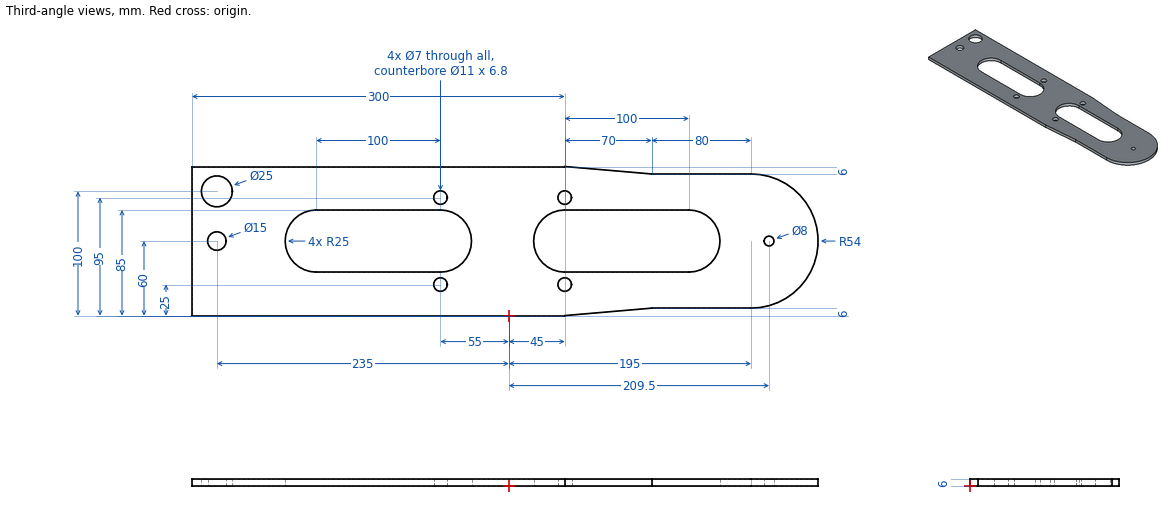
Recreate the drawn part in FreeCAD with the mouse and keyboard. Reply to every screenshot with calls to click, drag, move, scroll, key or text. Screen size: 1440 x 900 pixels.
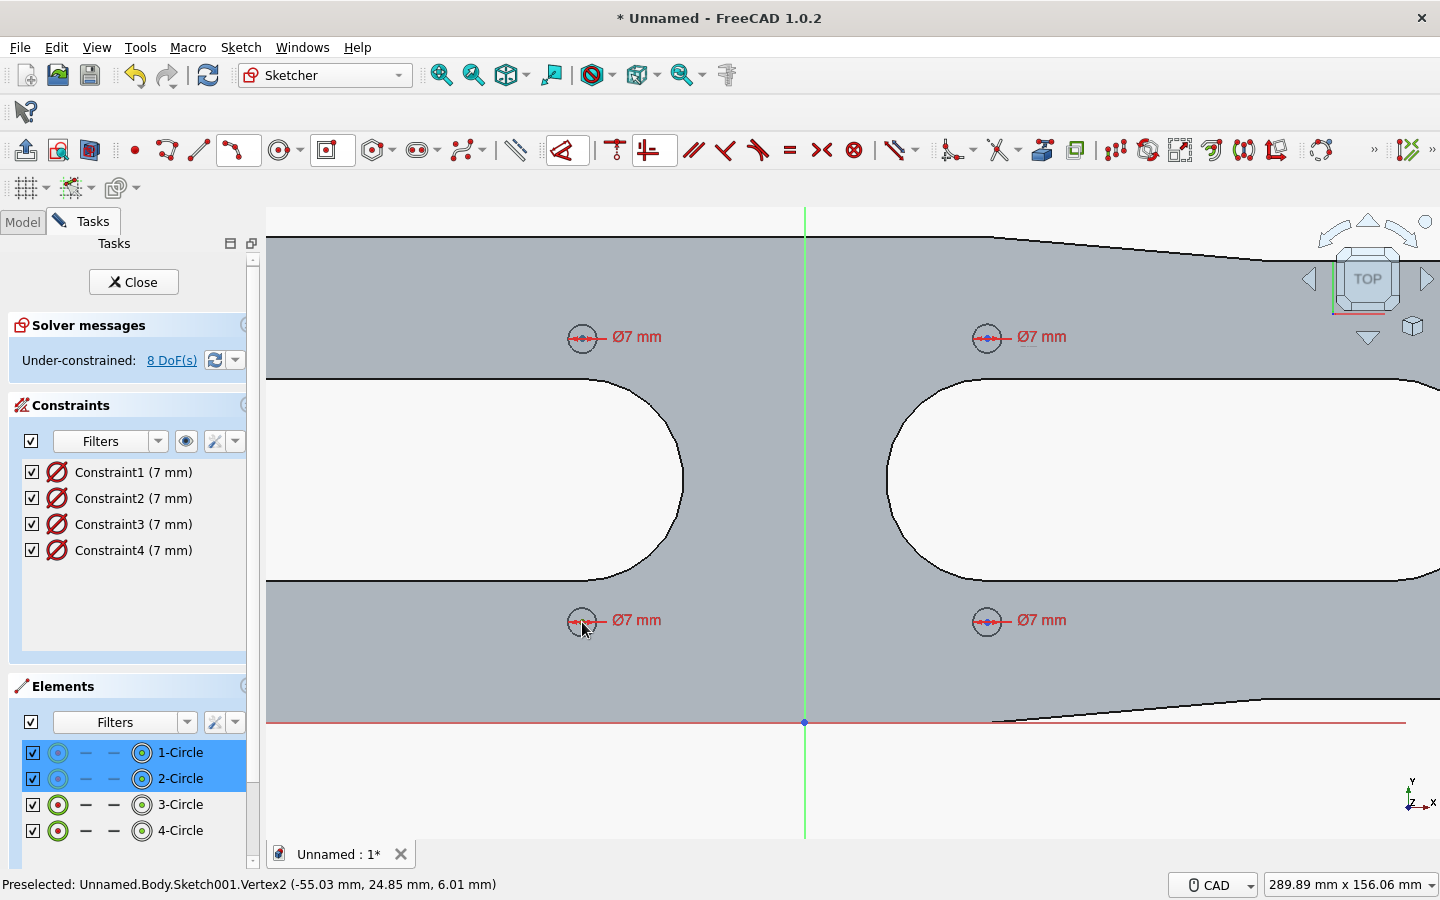
click(672, 150)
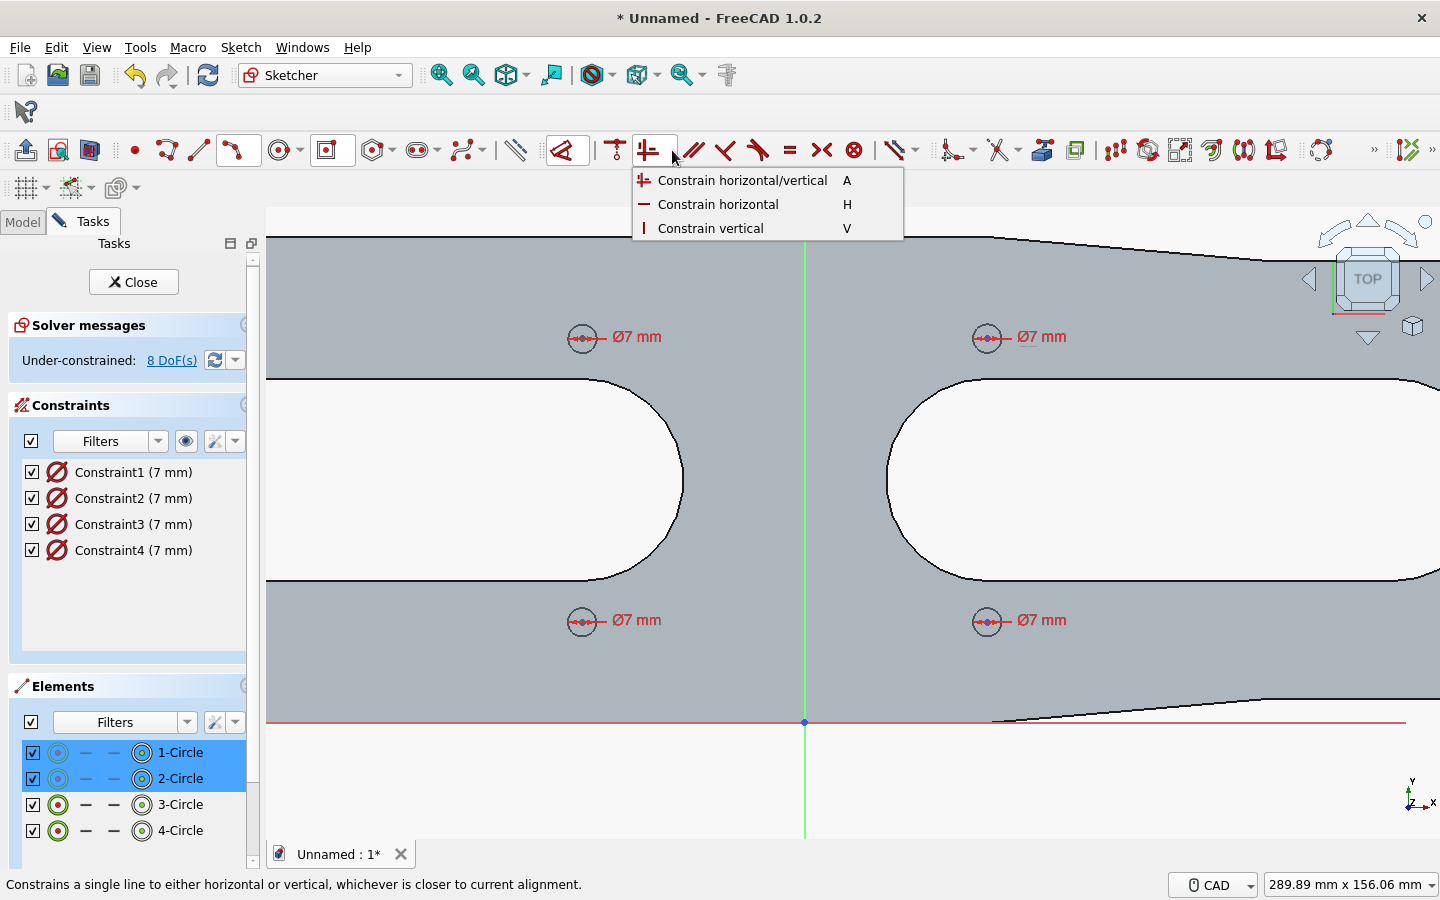
click(768, 228)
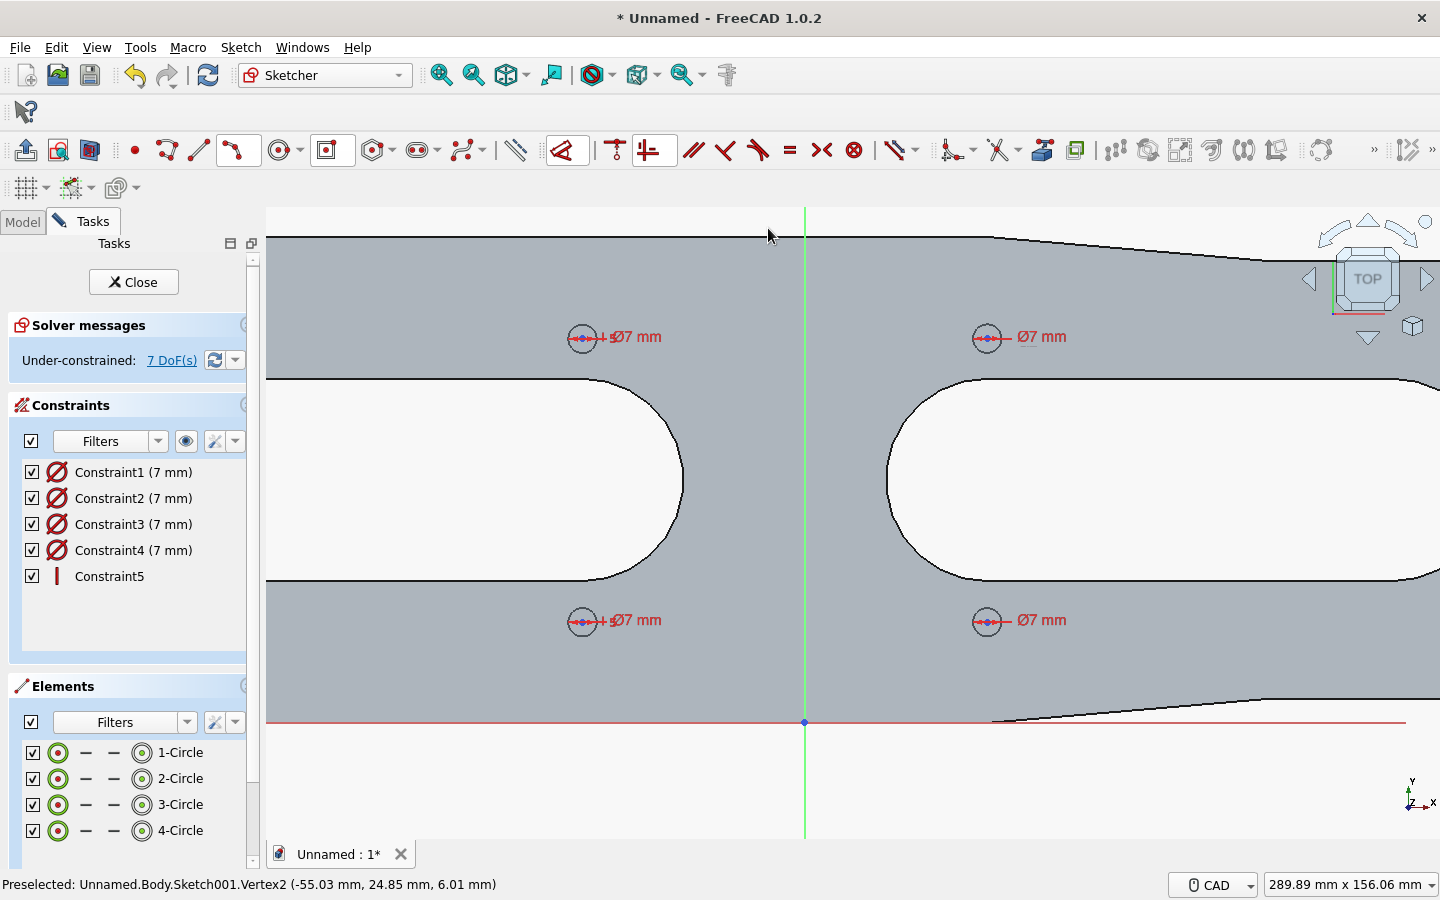
click(582, 339)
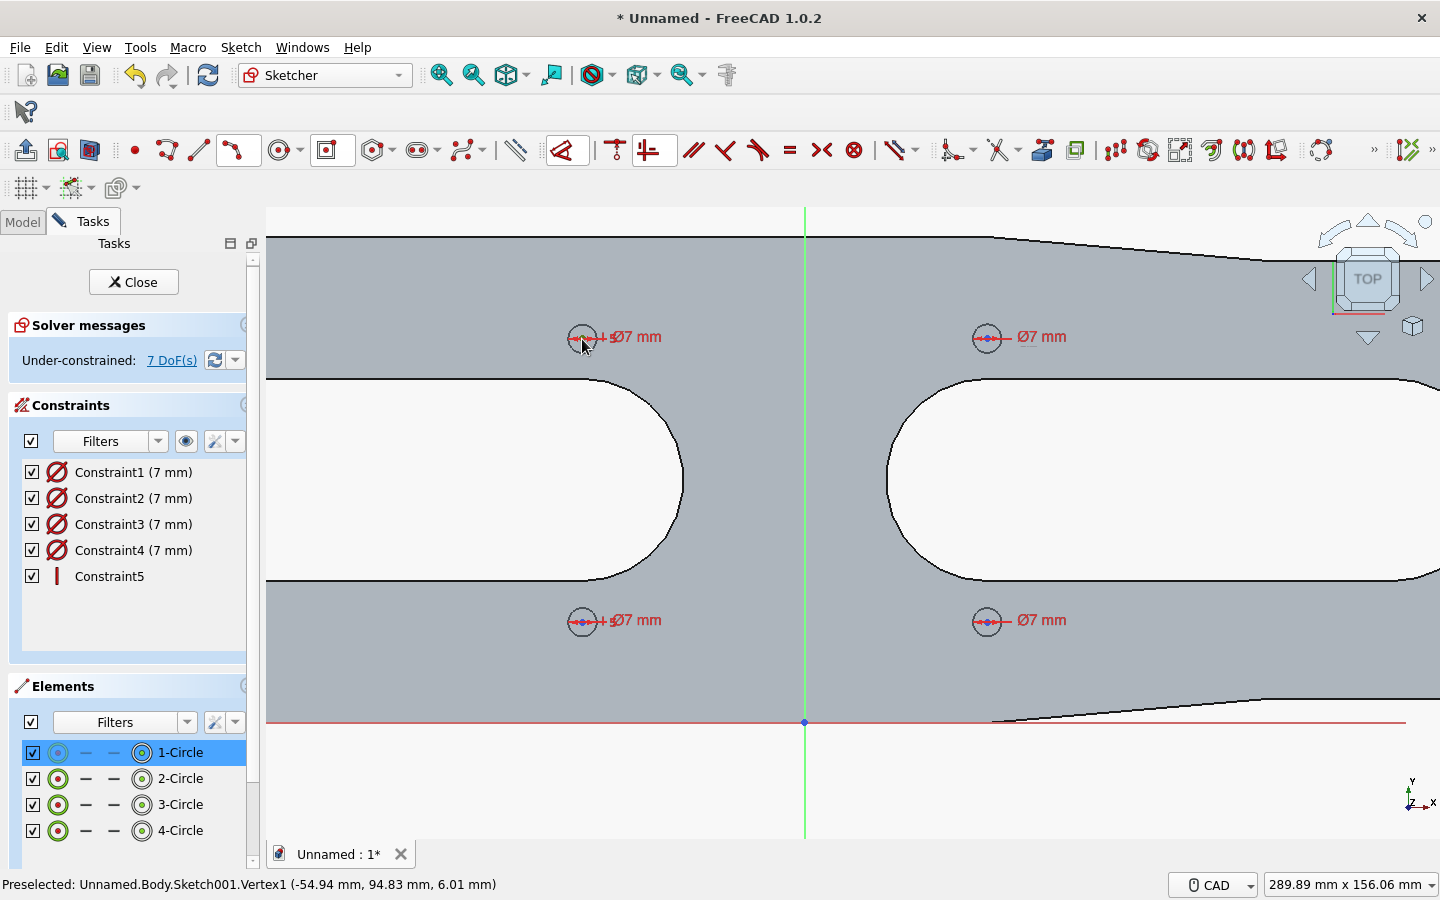
click(987, 339)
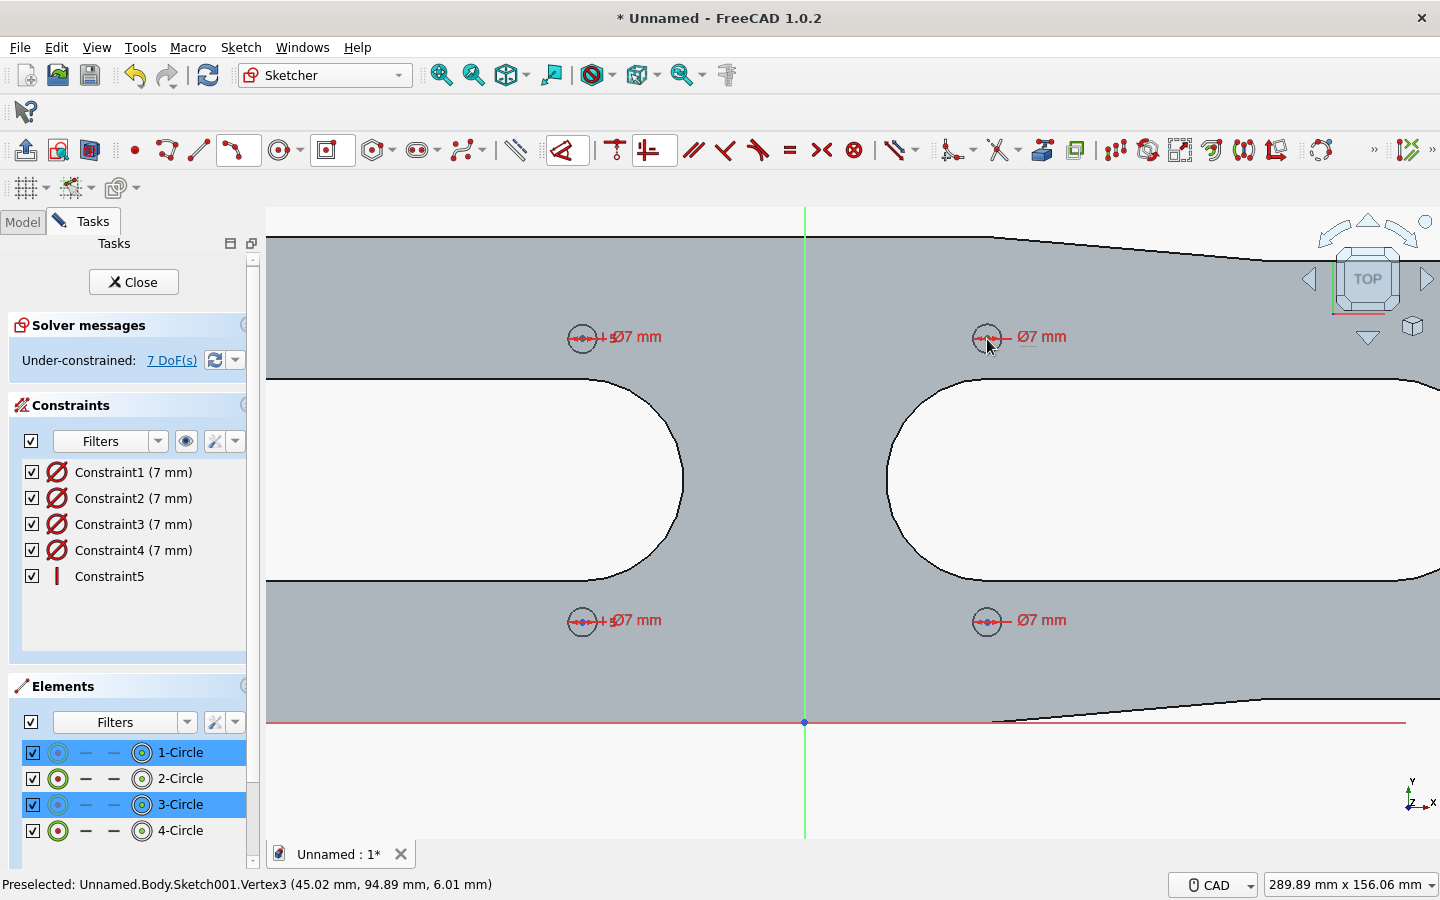
key(h)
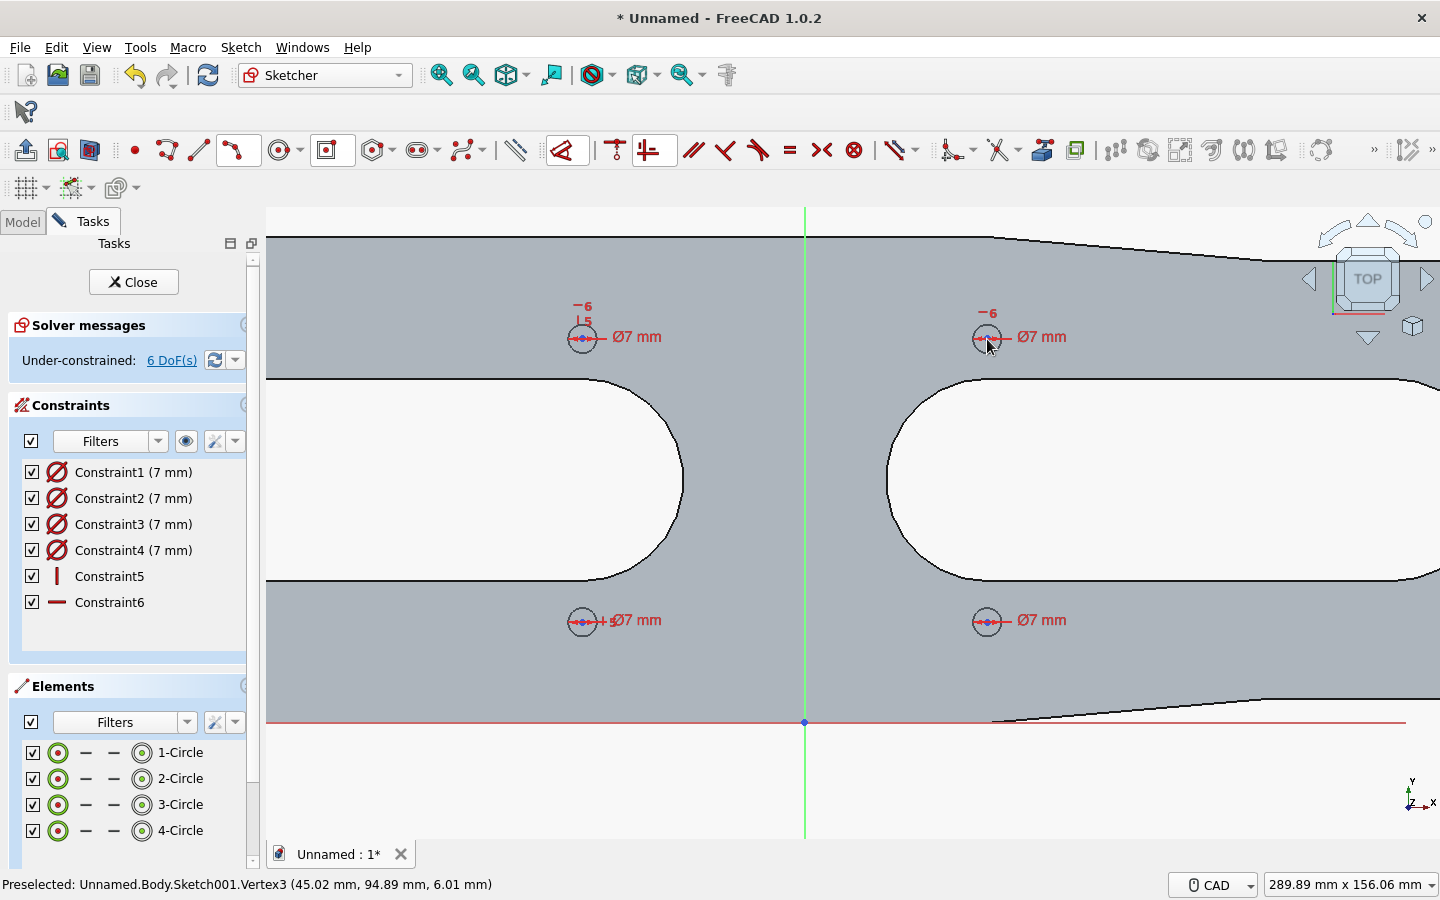
click(987, 339)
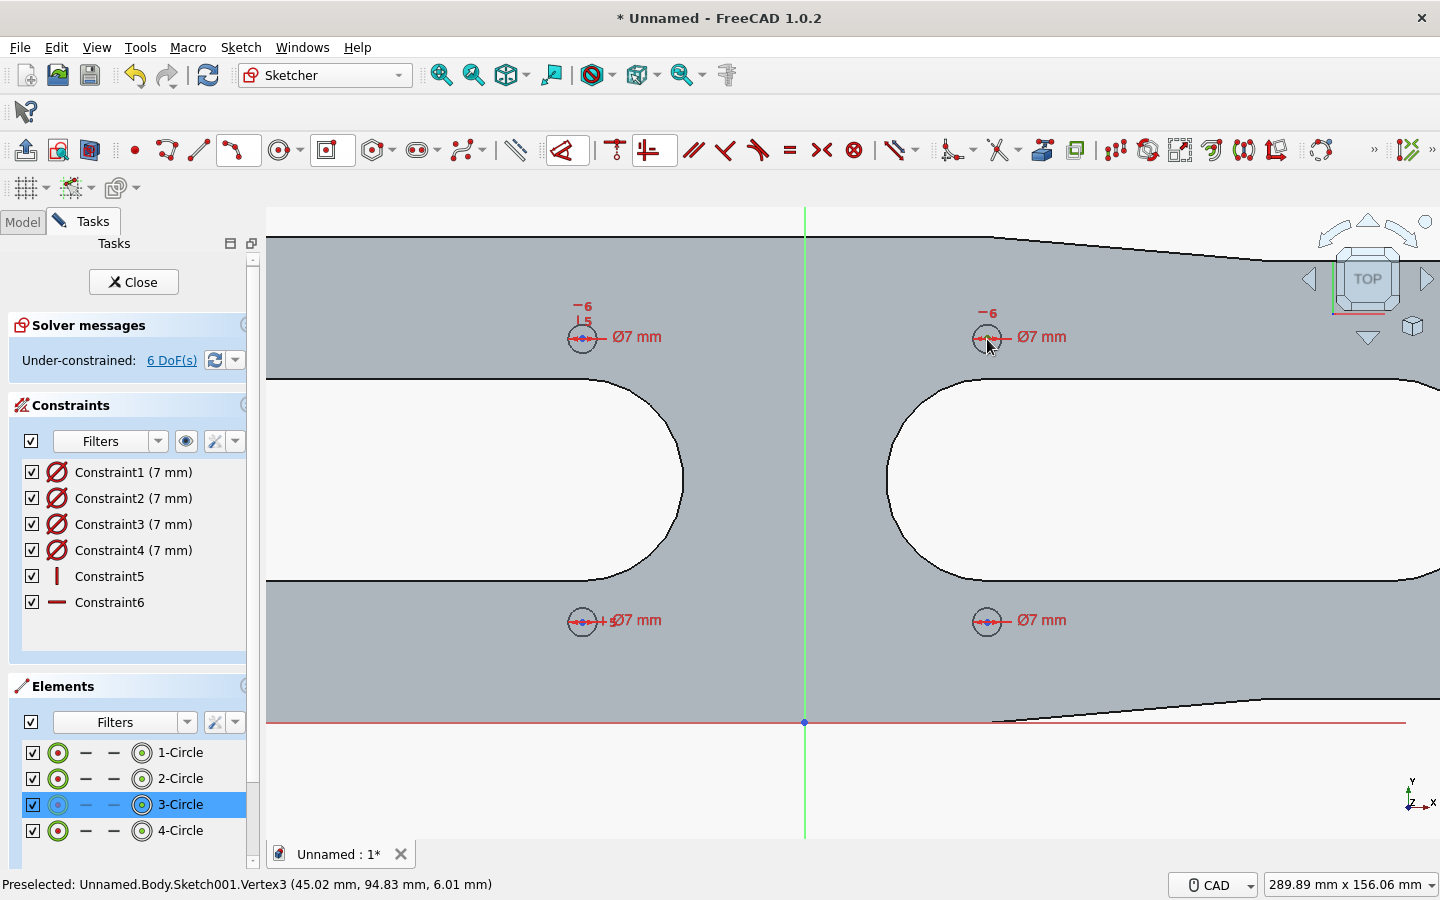
click(987, 622)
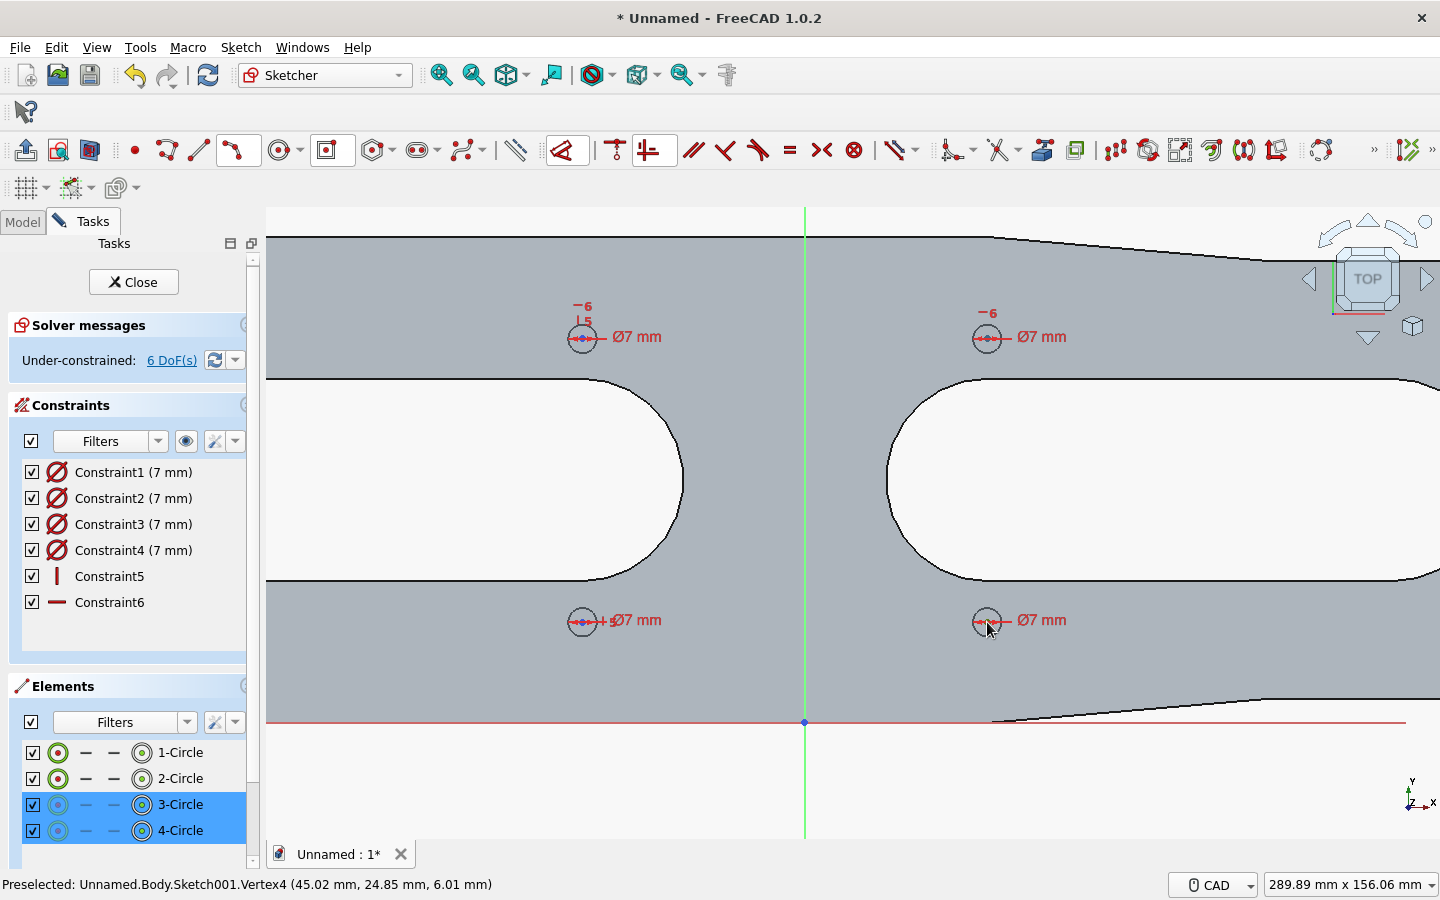
key(v)